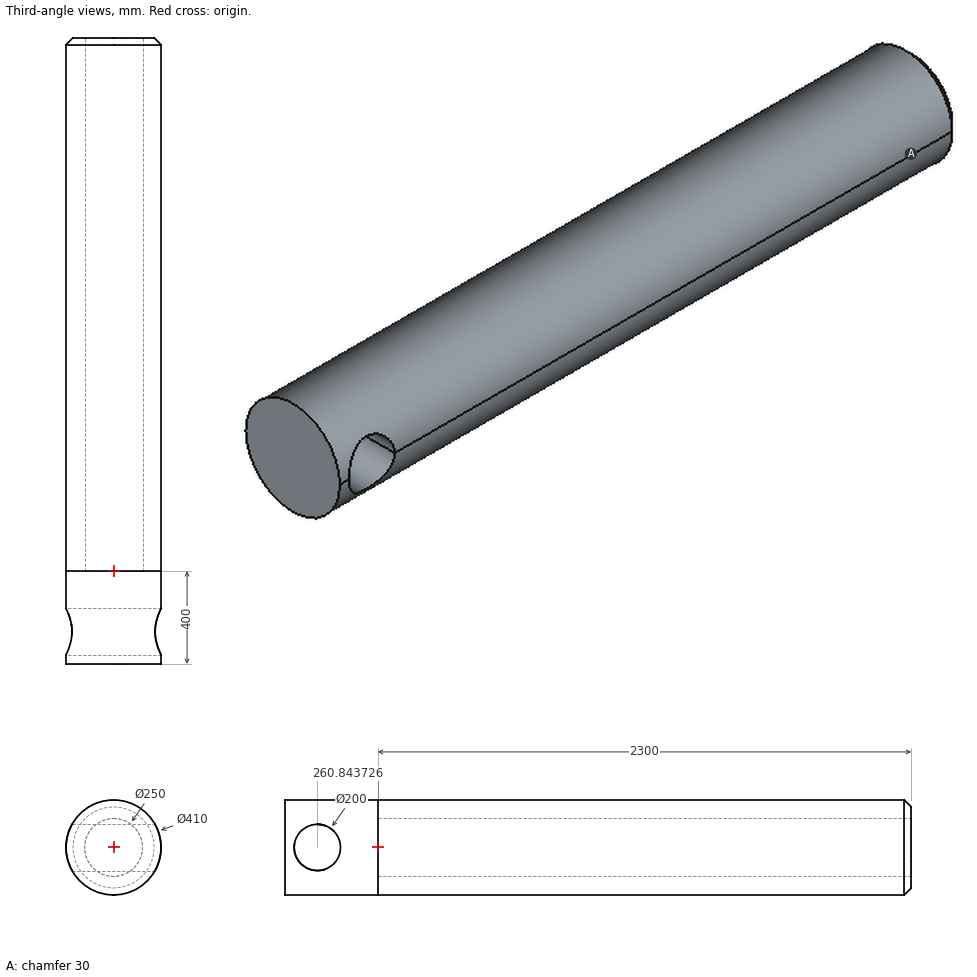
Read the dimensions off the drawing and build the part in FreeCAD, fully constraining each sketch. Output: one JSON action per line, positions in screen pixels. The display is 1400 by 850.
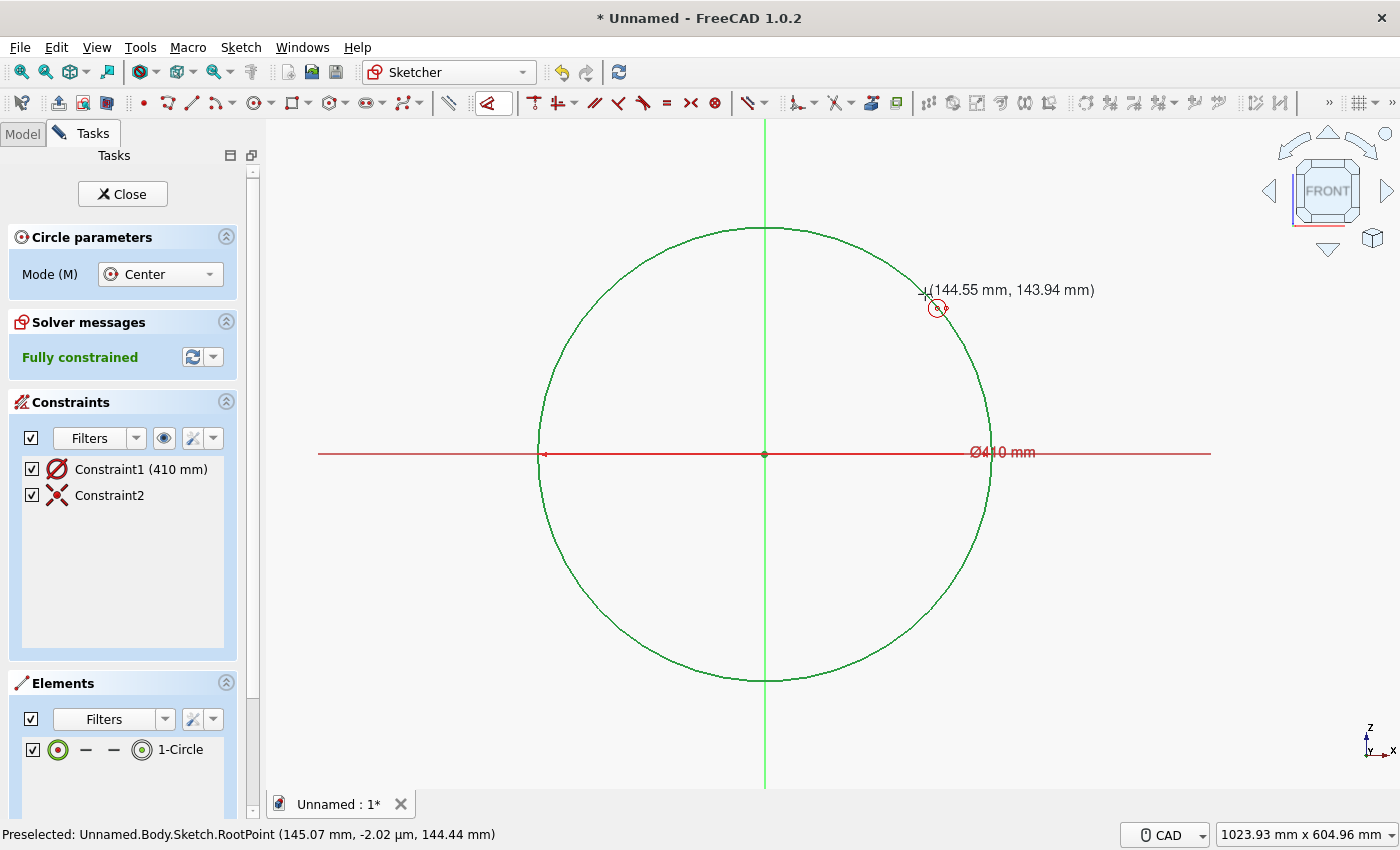
{"action": "left_click", "coordinate": [765, 454]}
{"action": "mouse_move", "coordinate": [863, 357]}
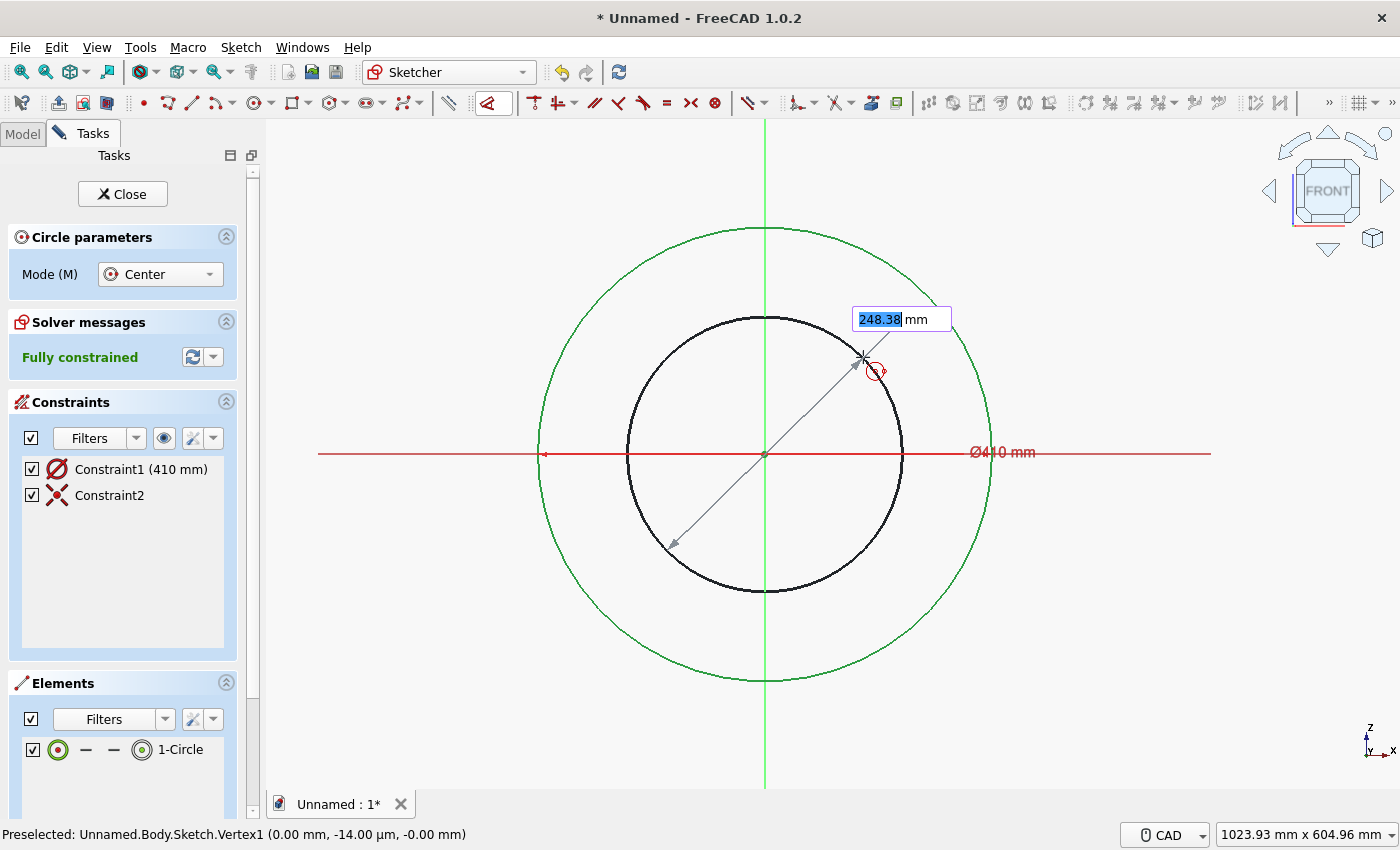
{"action": "type", "text": "250"}
{"action": "key", "text": "Return"}
{"action": "key", "text": "Escape"}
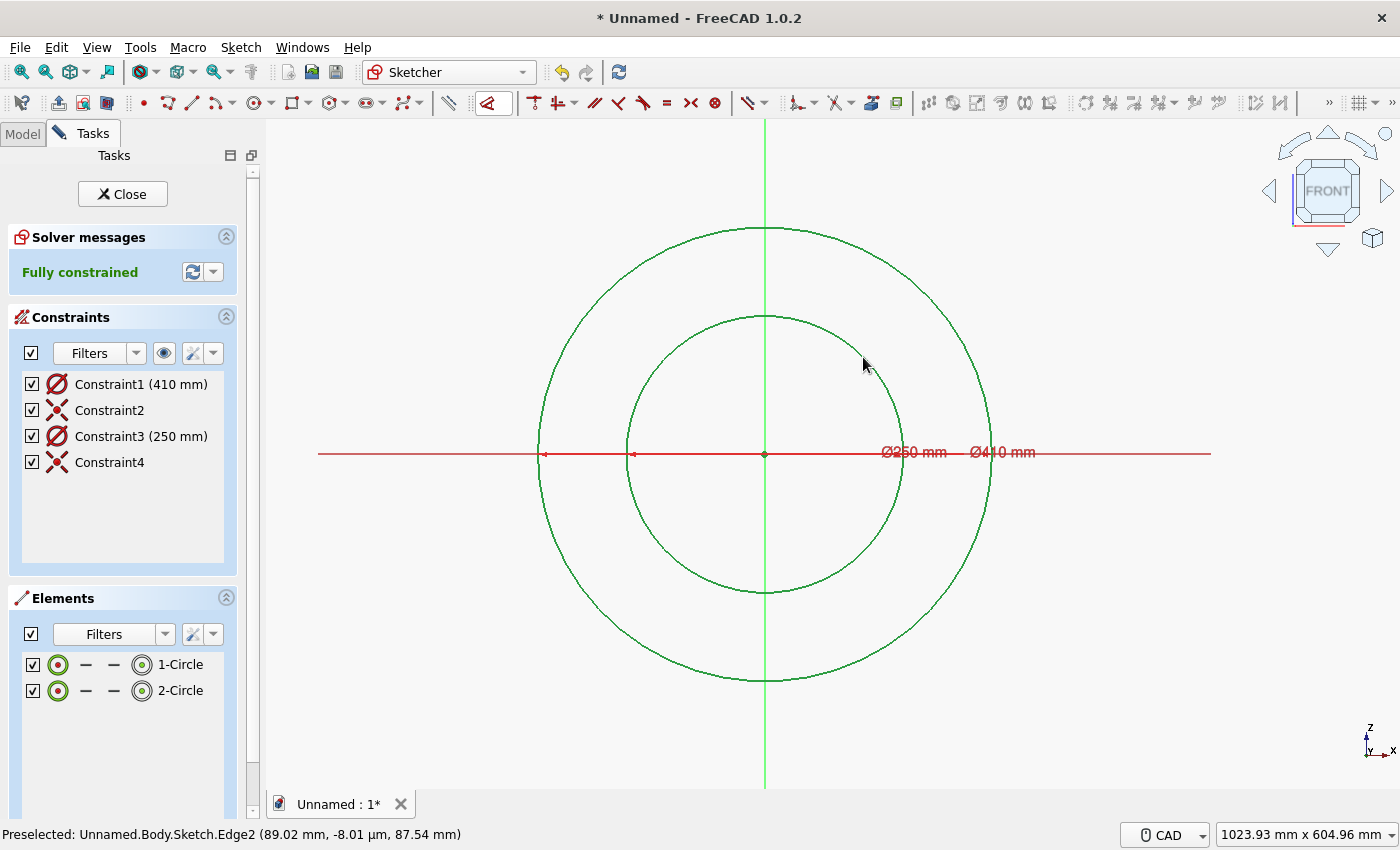
{"action": "left_click", "coordinate": [123, 194]}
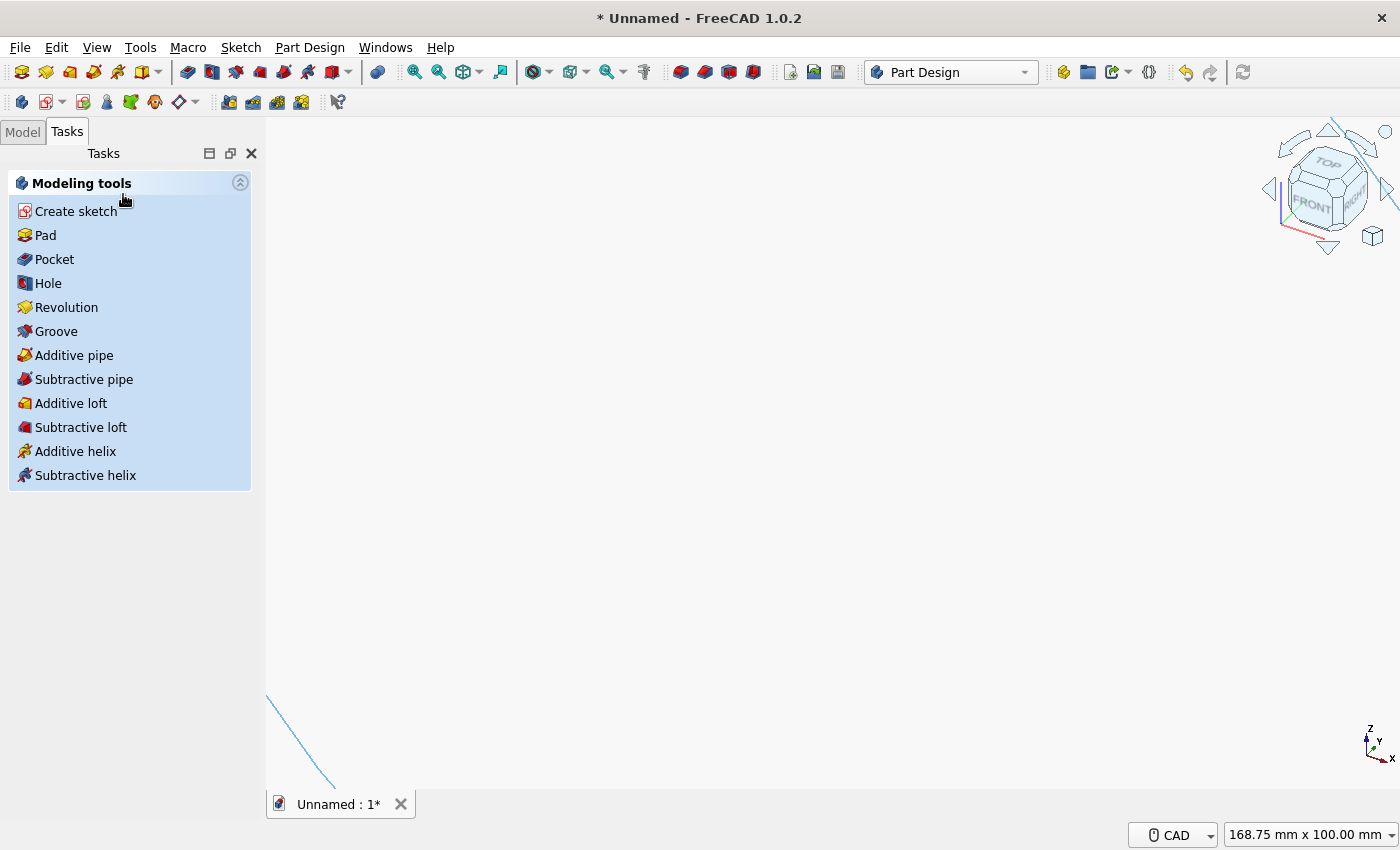
{"action": "left_click", "coordinate": [22, 72]}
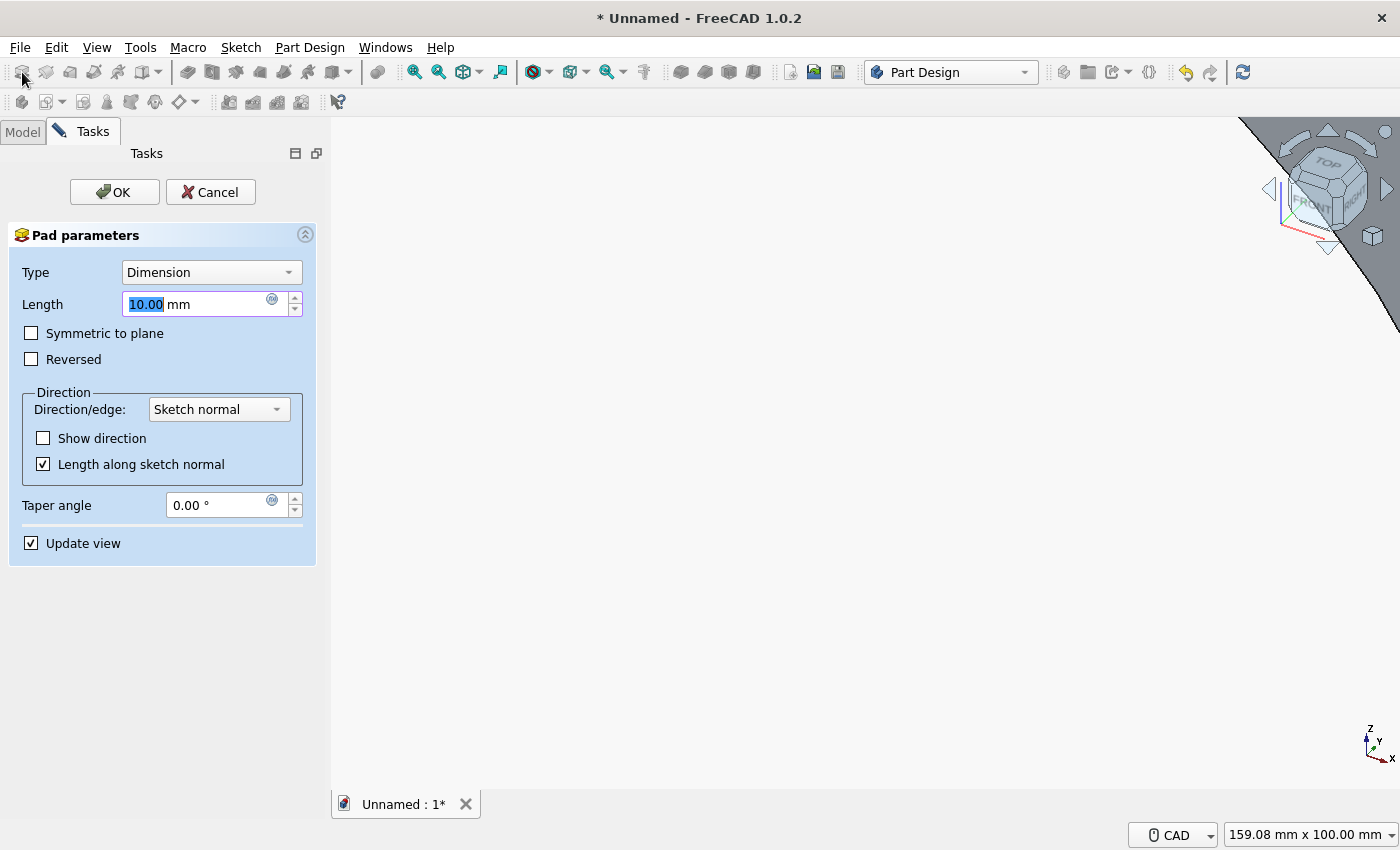
{"action": "type", "text": "2300"}
{"action": "key", "text": "Tab"}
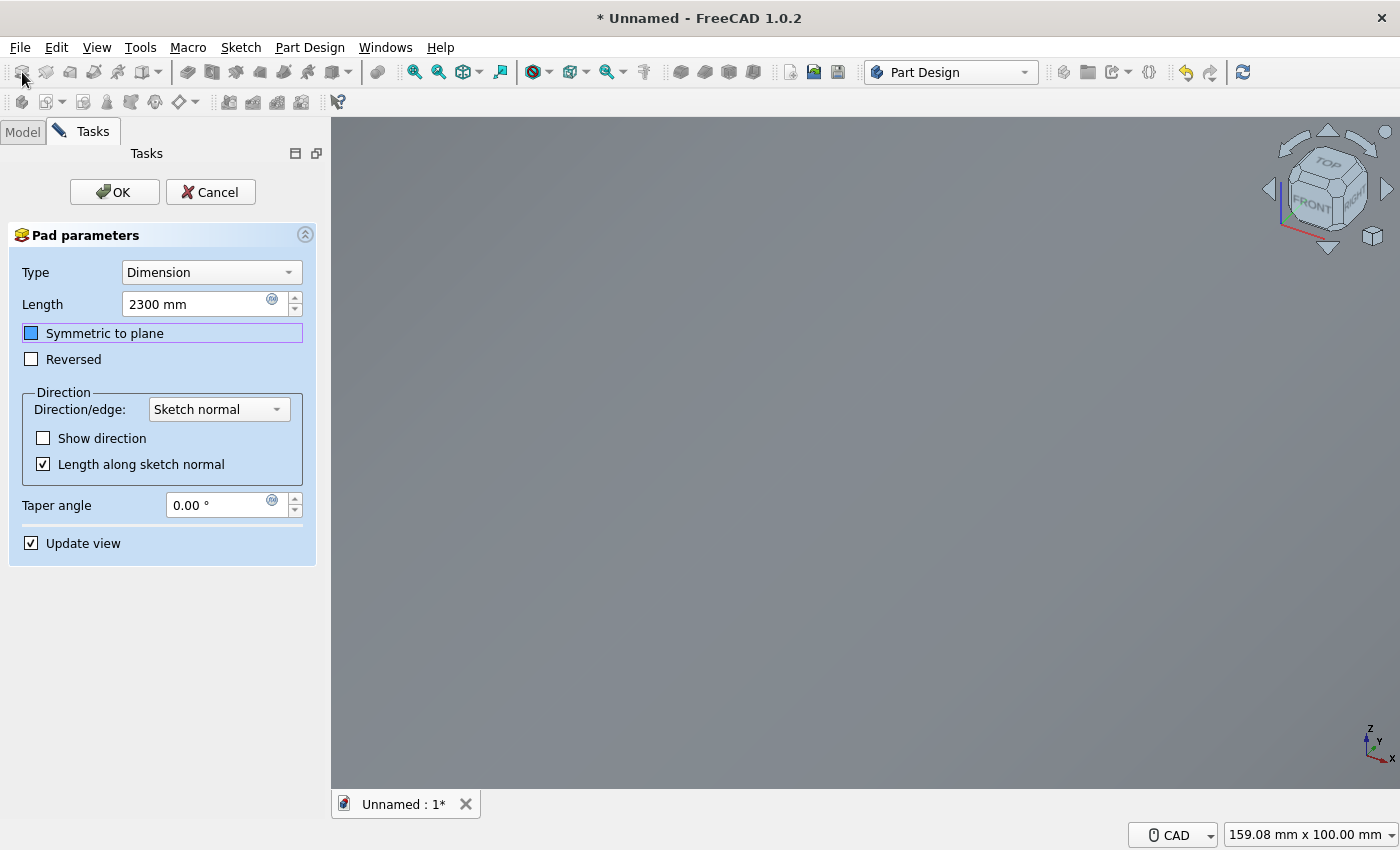
{"action": "left_click", "coordinate": [30, 359]}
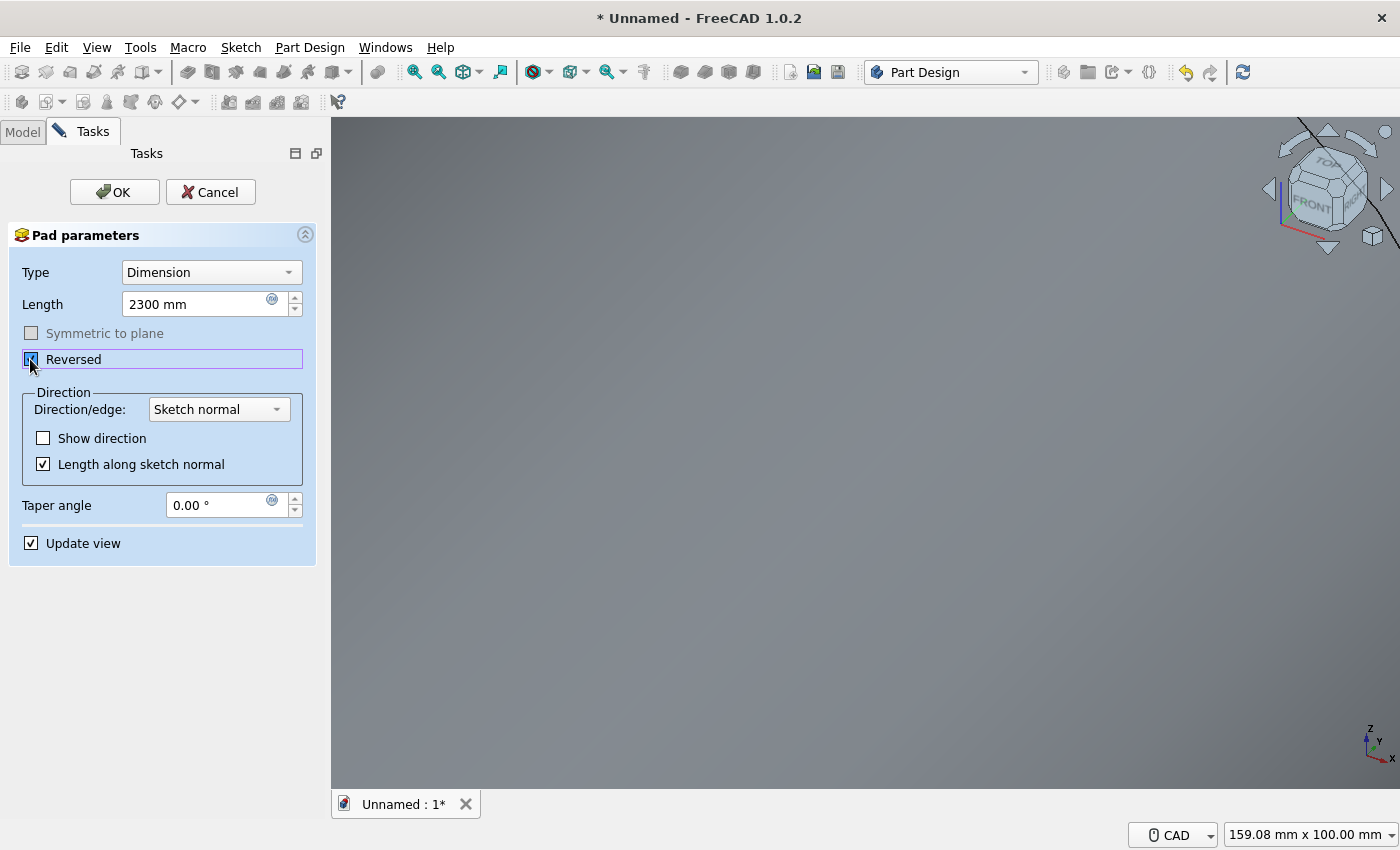
{"action": "left_click", "coordinate": [115, 192]}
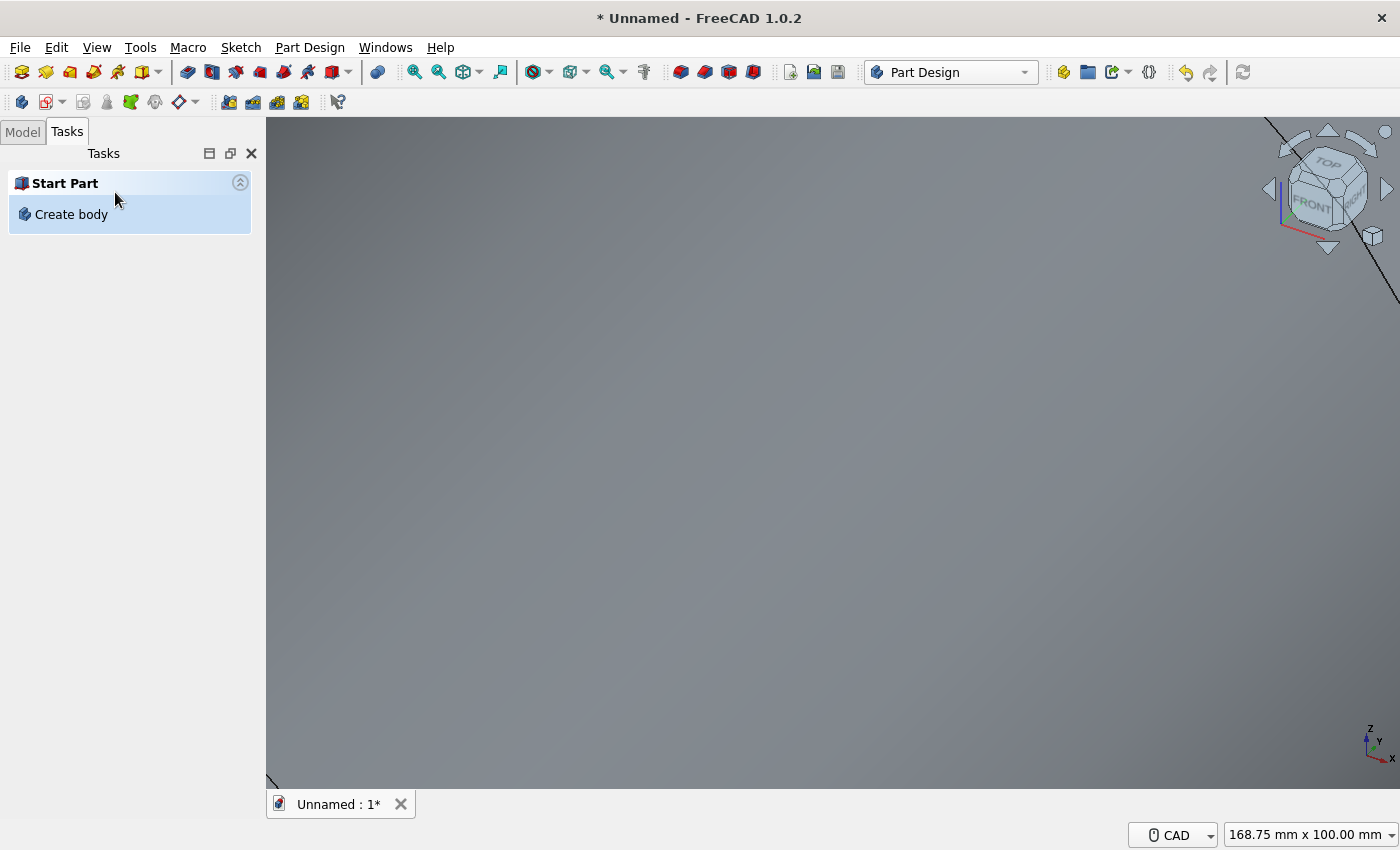
{"action": "left_click", "coordinate": [416, 72]}